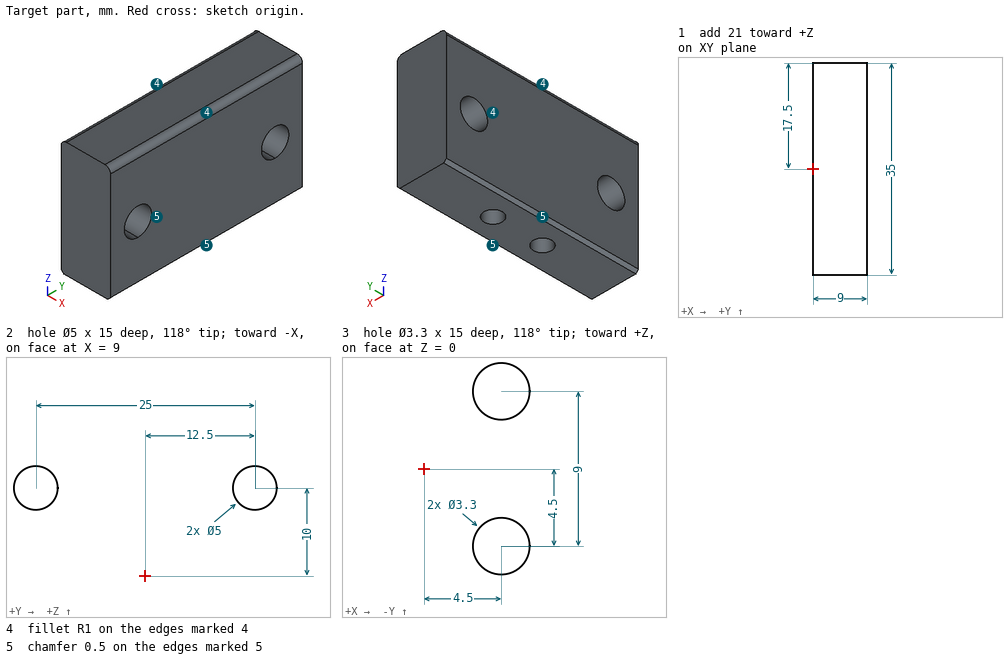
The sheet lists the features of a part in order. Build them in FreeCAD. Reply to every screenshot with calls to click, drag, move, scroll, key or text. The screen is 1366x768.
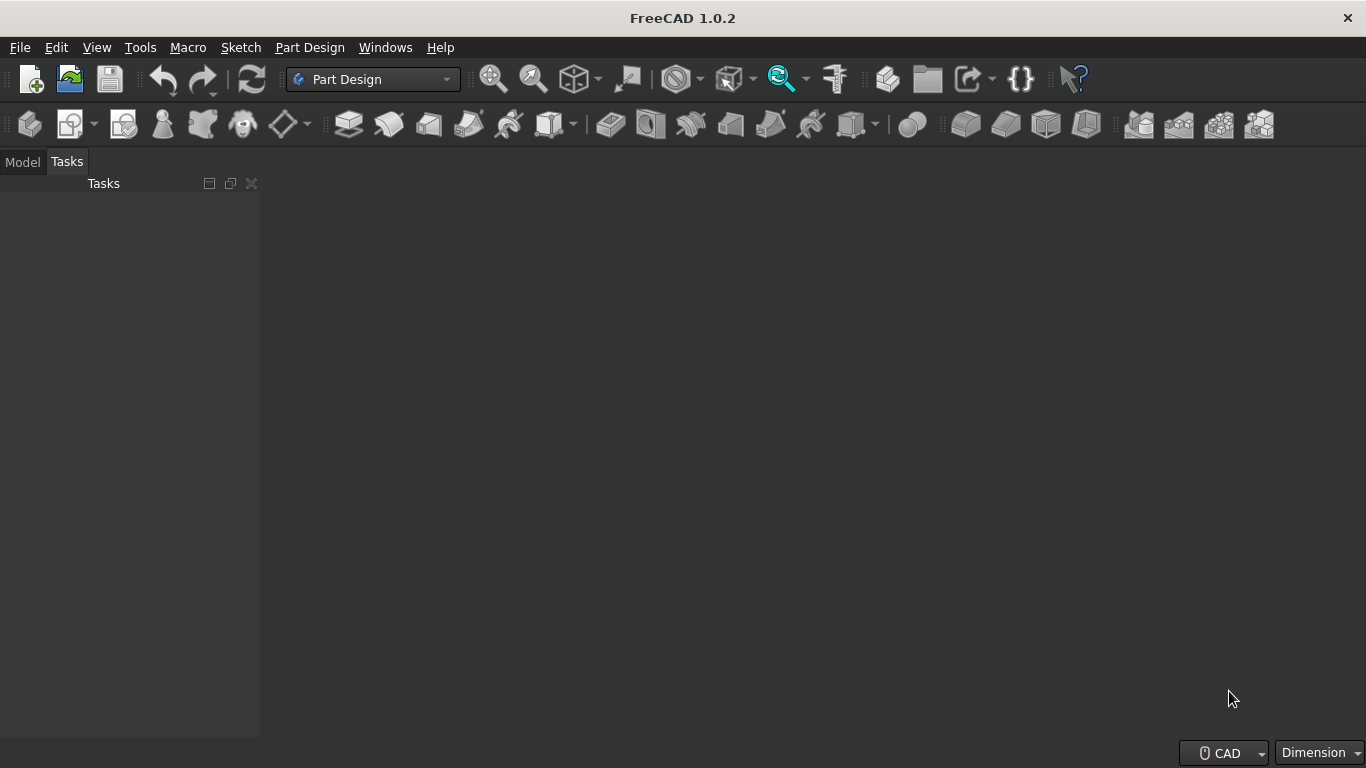
key(ctrl+n)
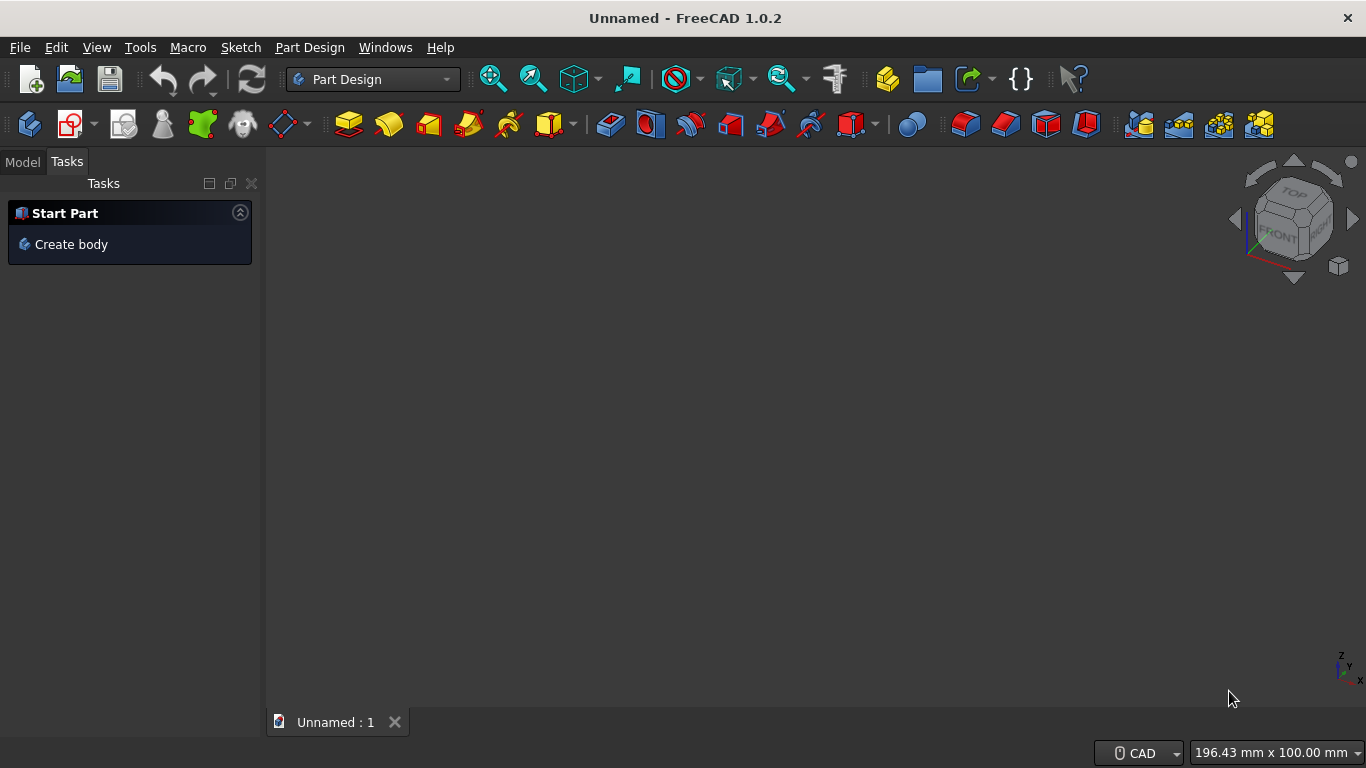
click(70, 124)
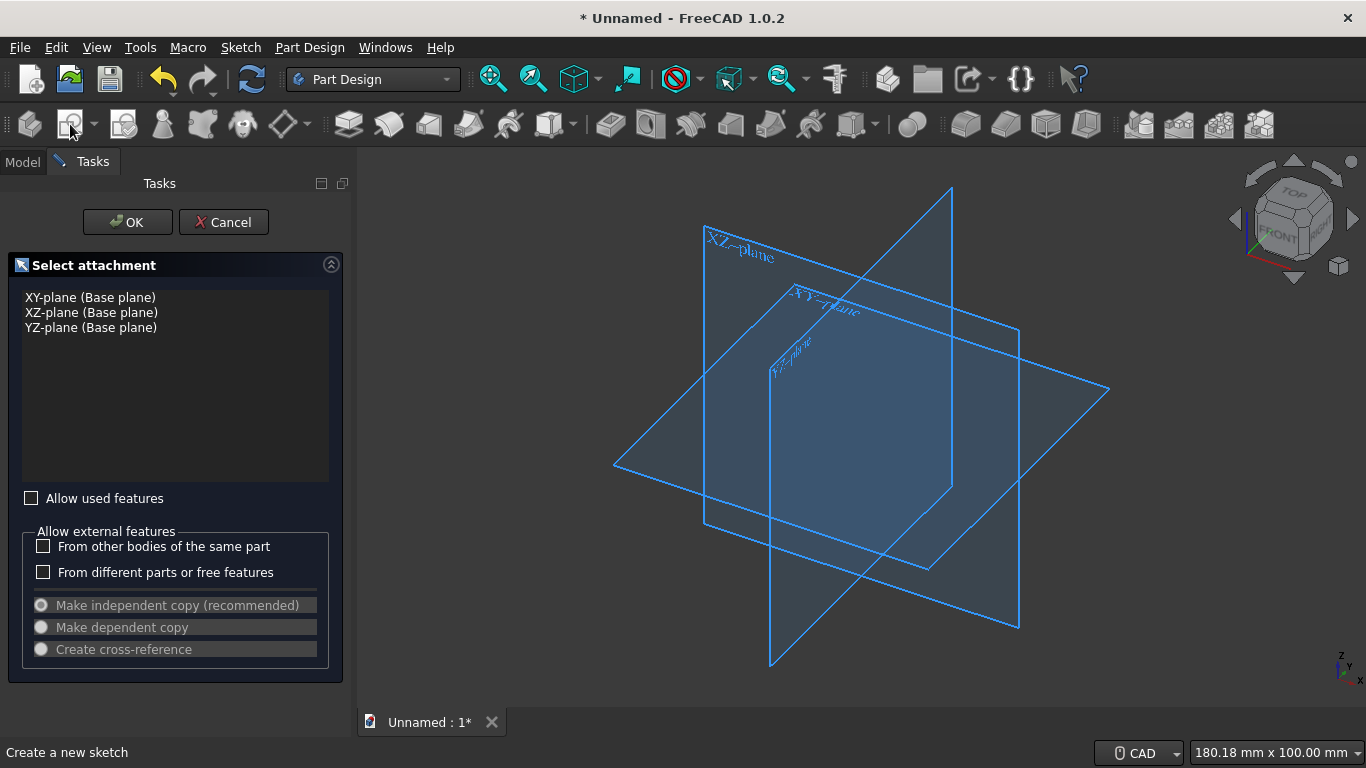
click(82, 298)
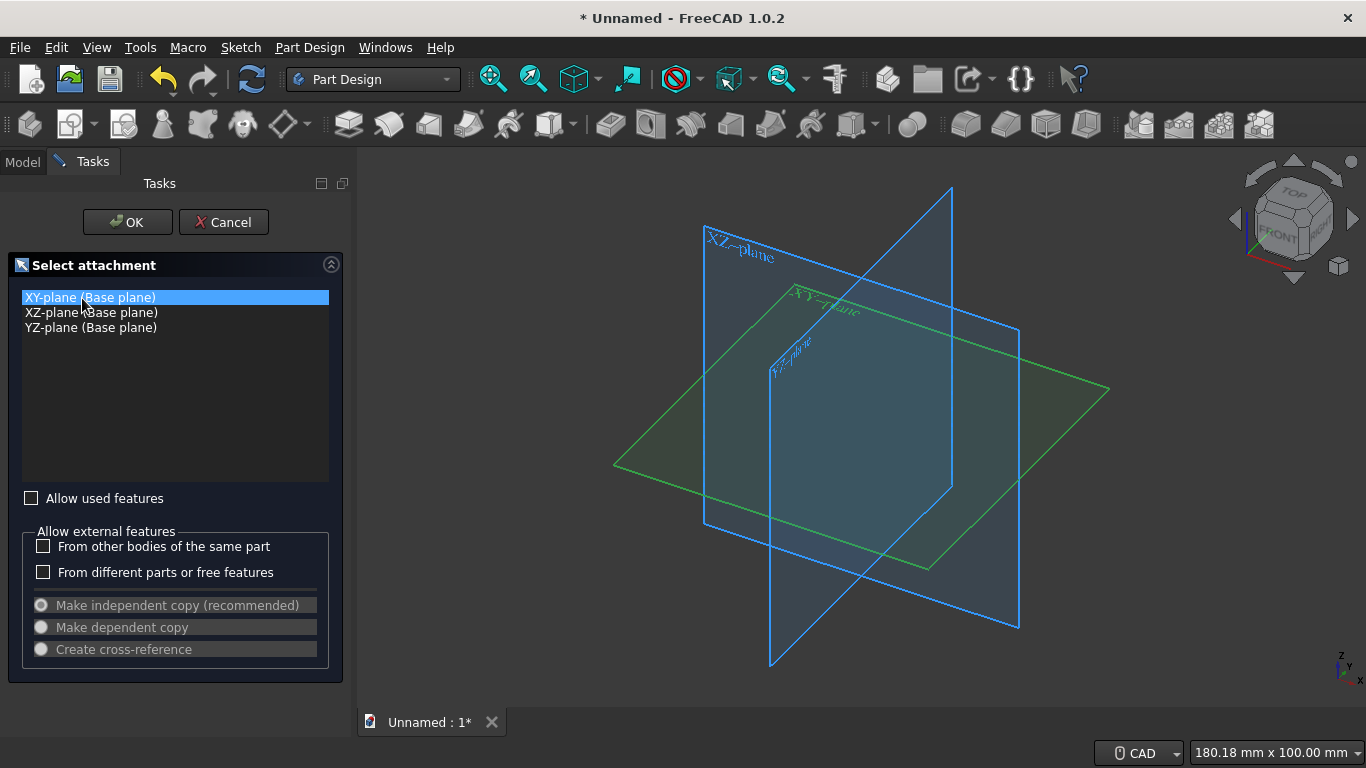
click(128, 222)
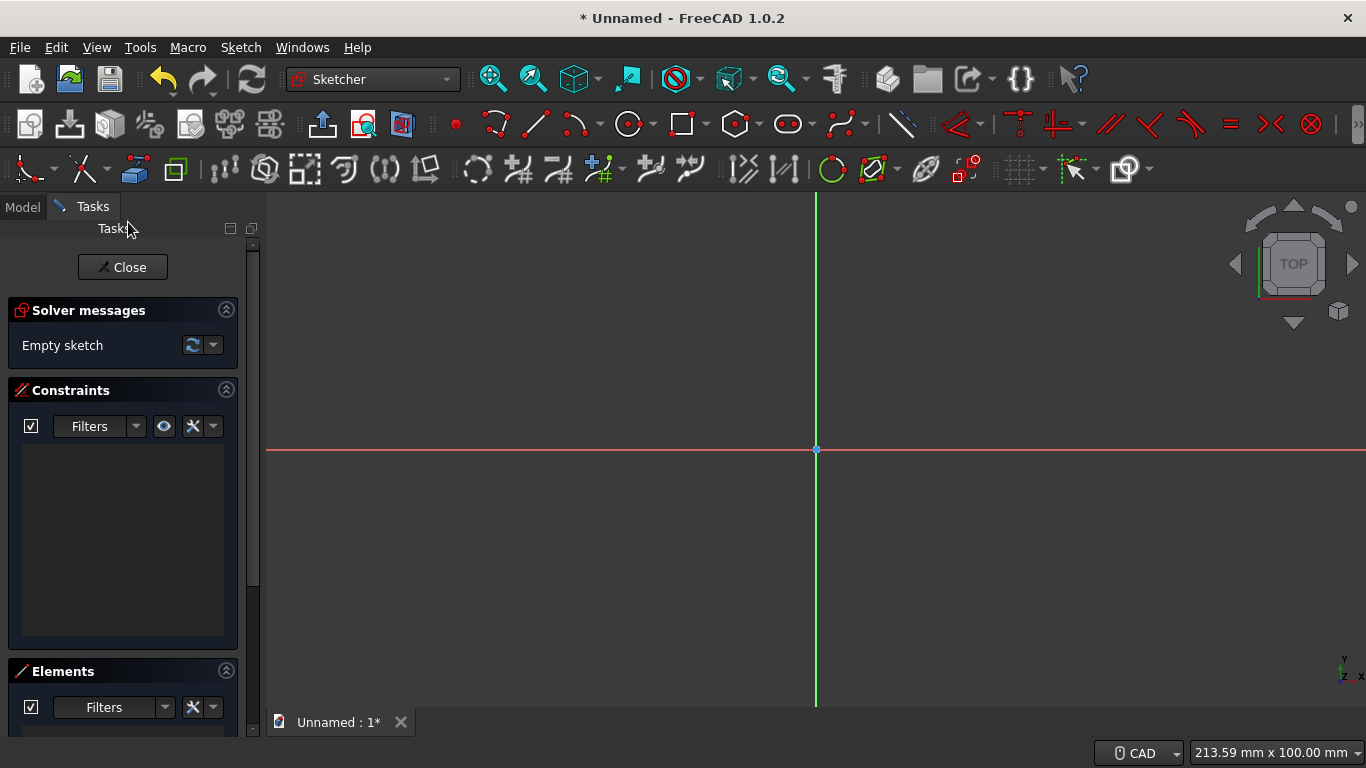
scroll(951, 449, up, 3)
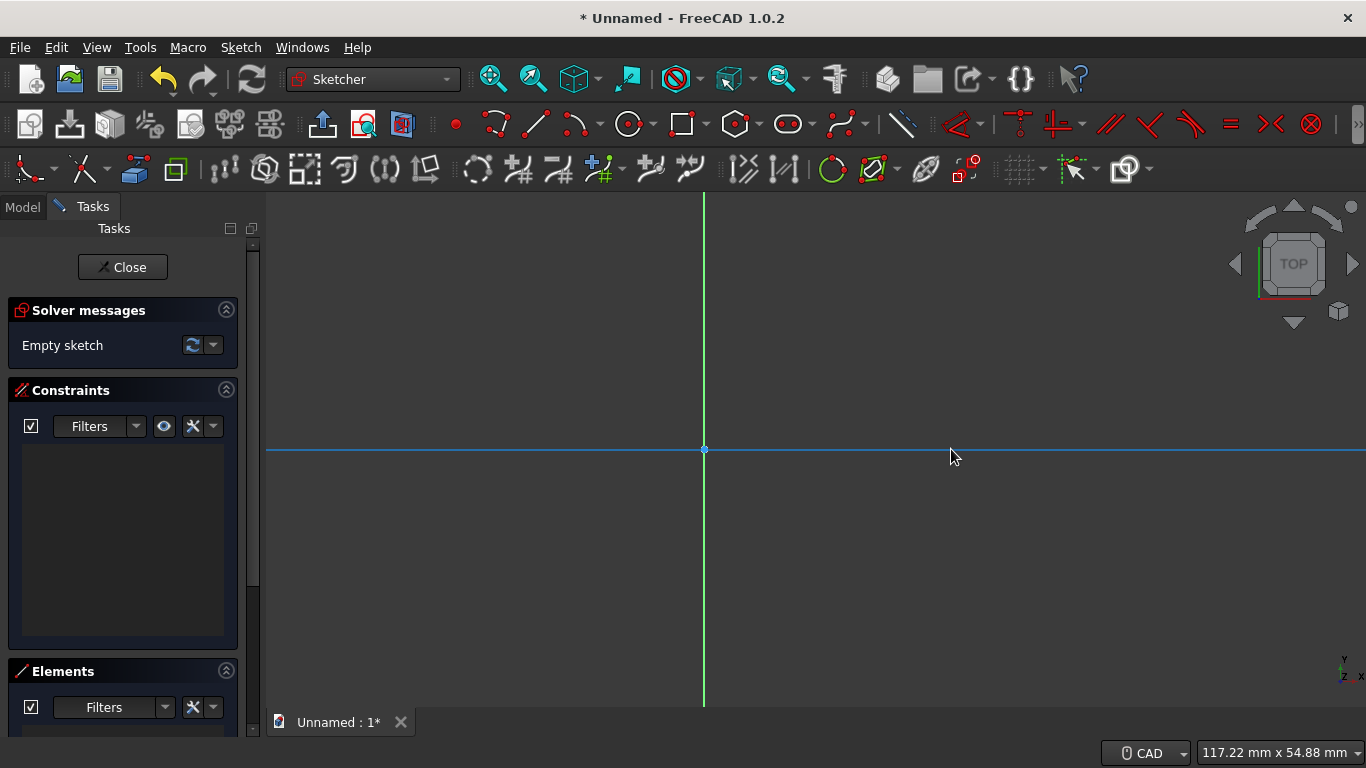
click(682, 124)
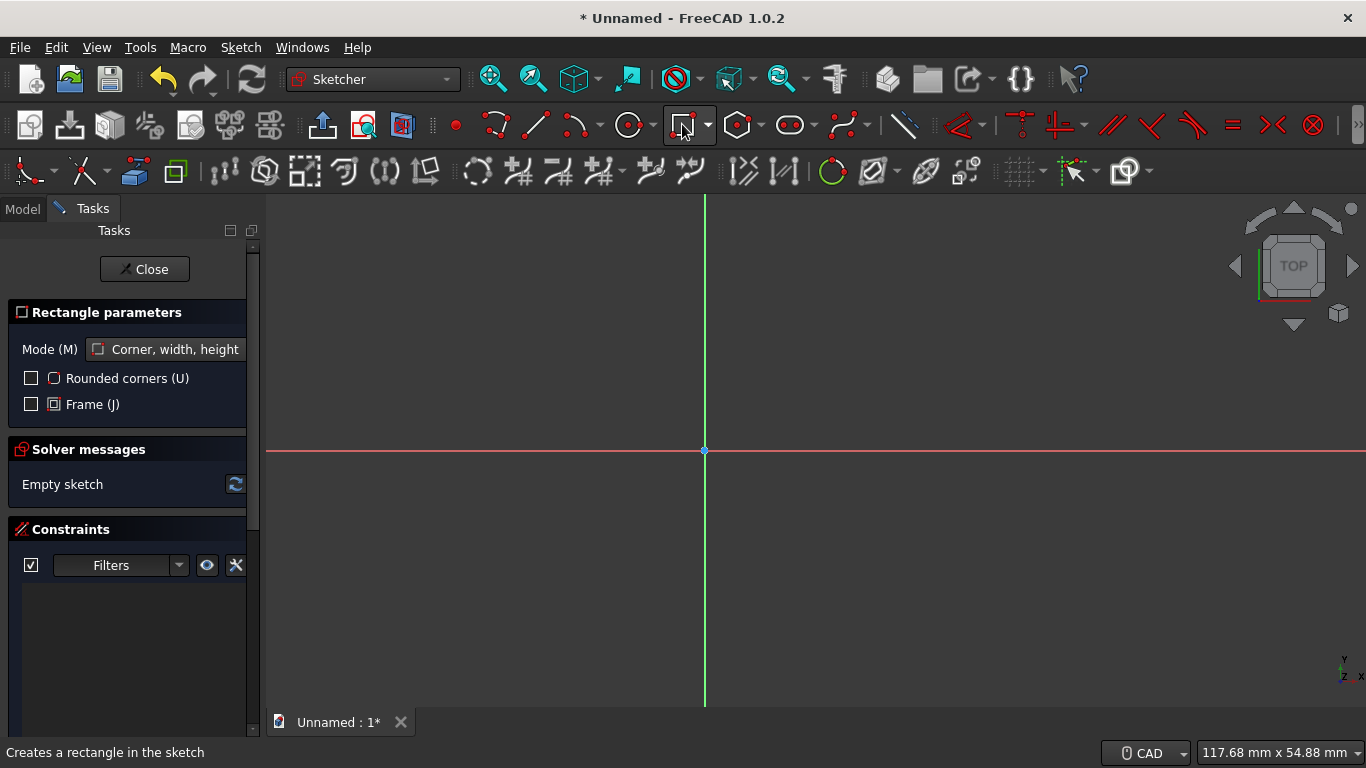
click(705, 287)
move(789, 614)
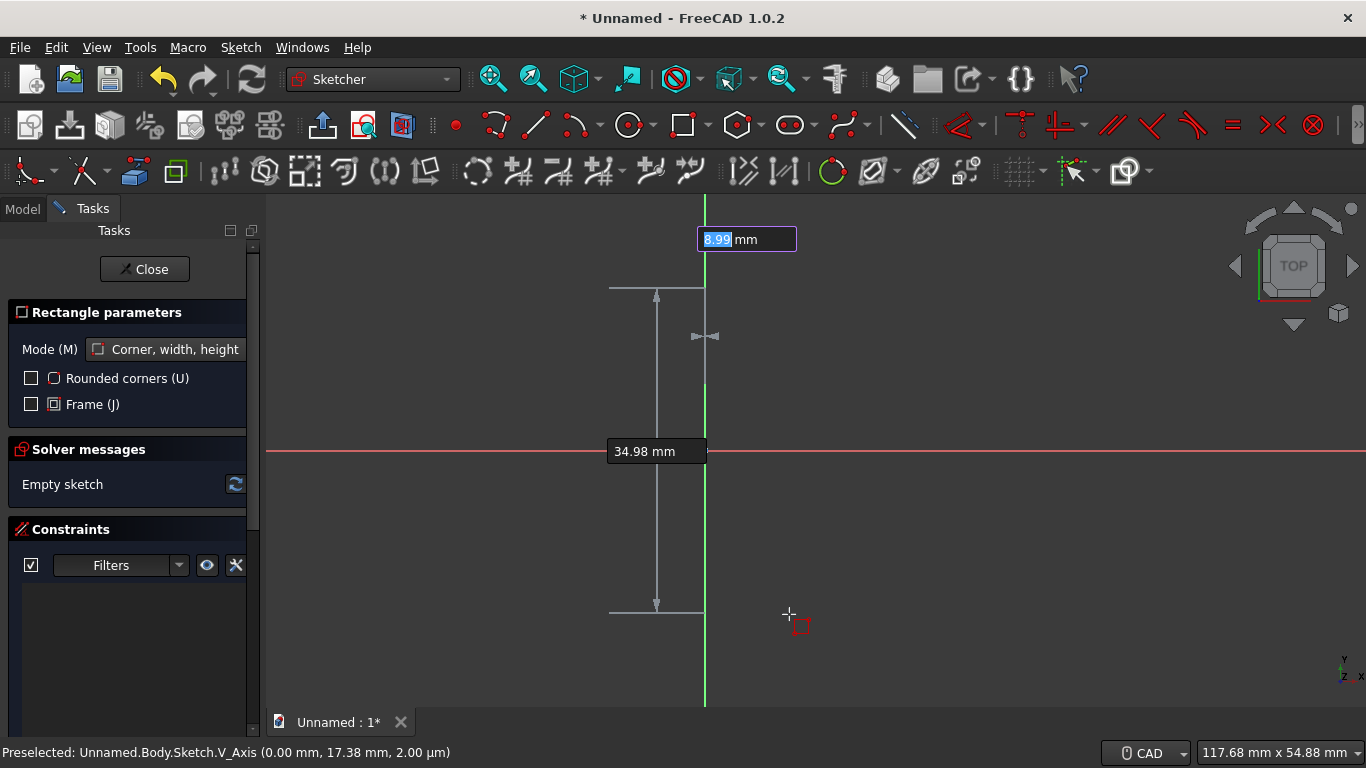
text(9)
key(Tab)
text(35)
key(Return)
key(Escape)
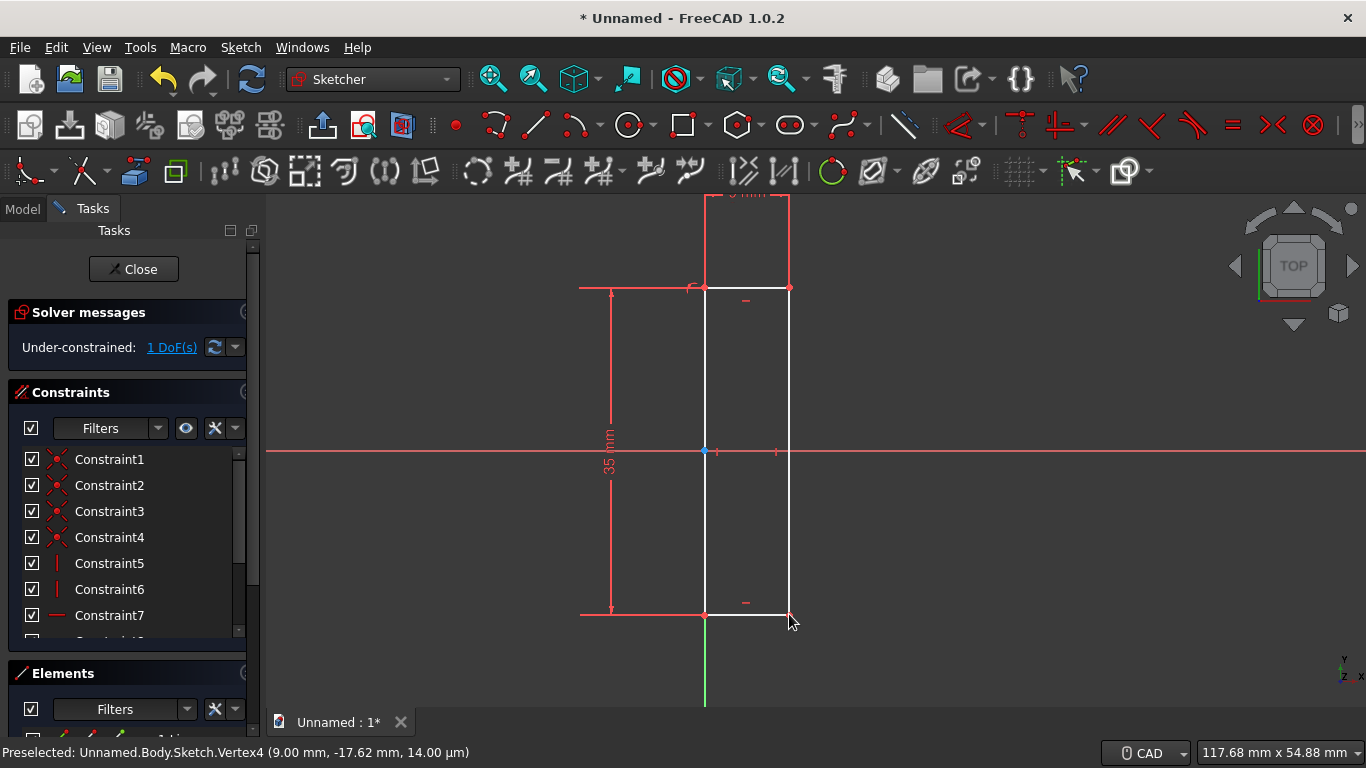
click(705, 288)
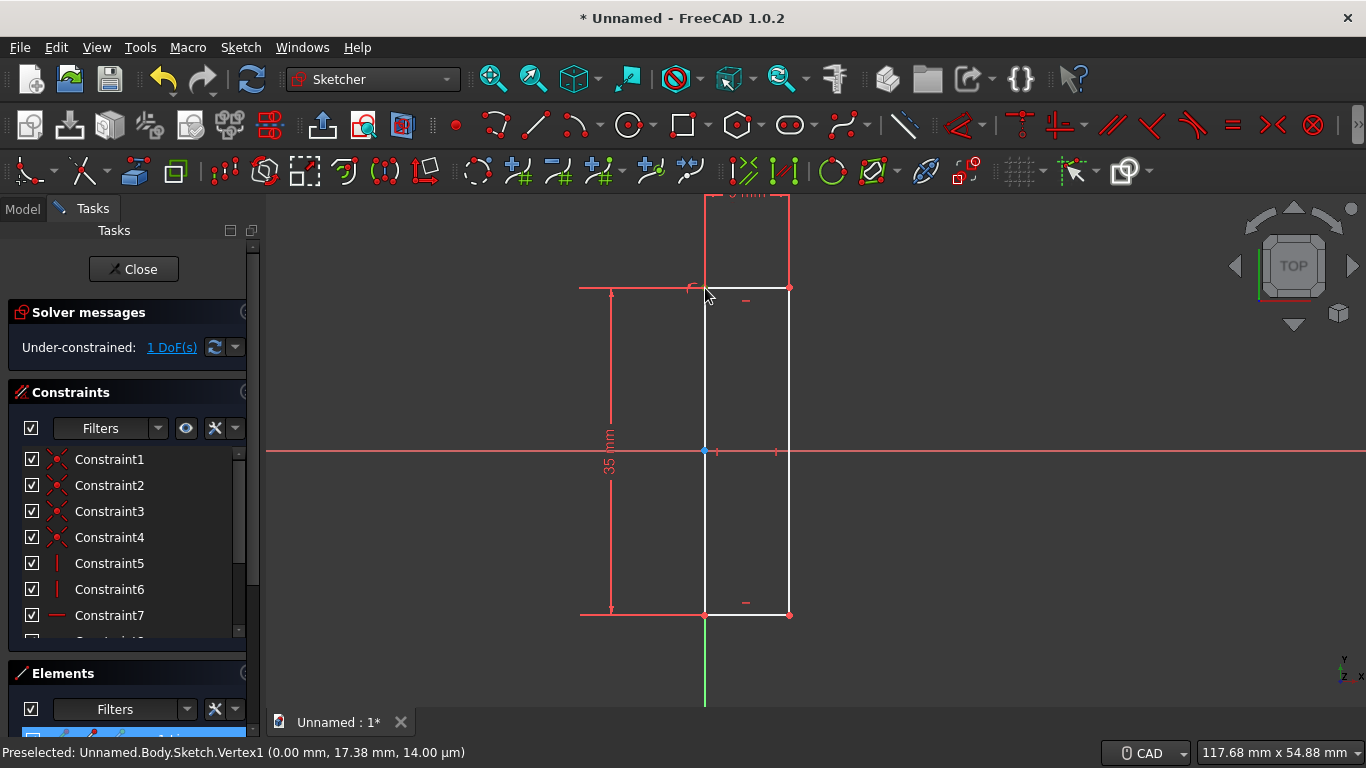
click(984, 126)